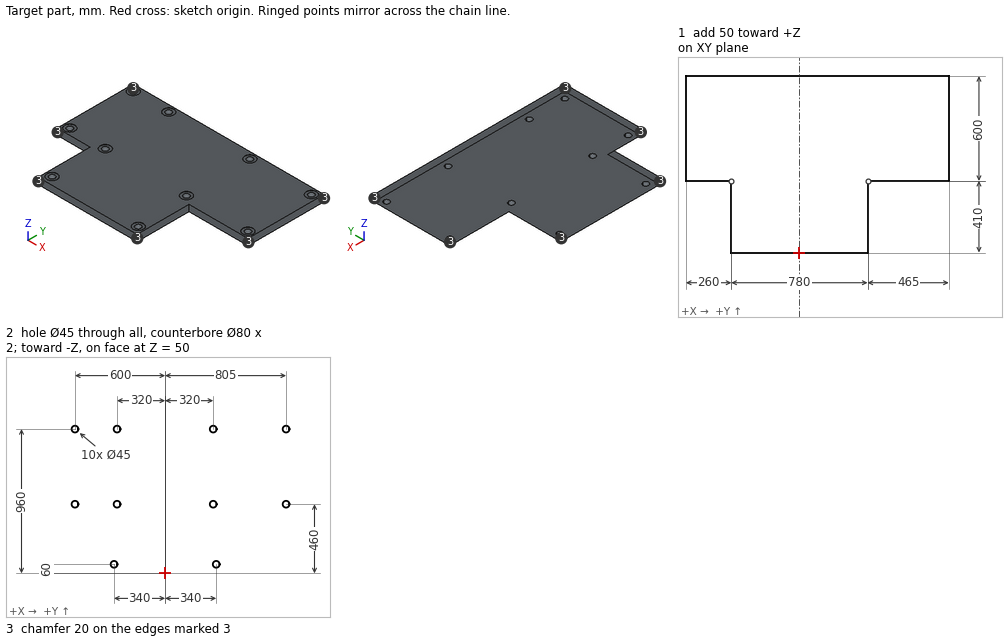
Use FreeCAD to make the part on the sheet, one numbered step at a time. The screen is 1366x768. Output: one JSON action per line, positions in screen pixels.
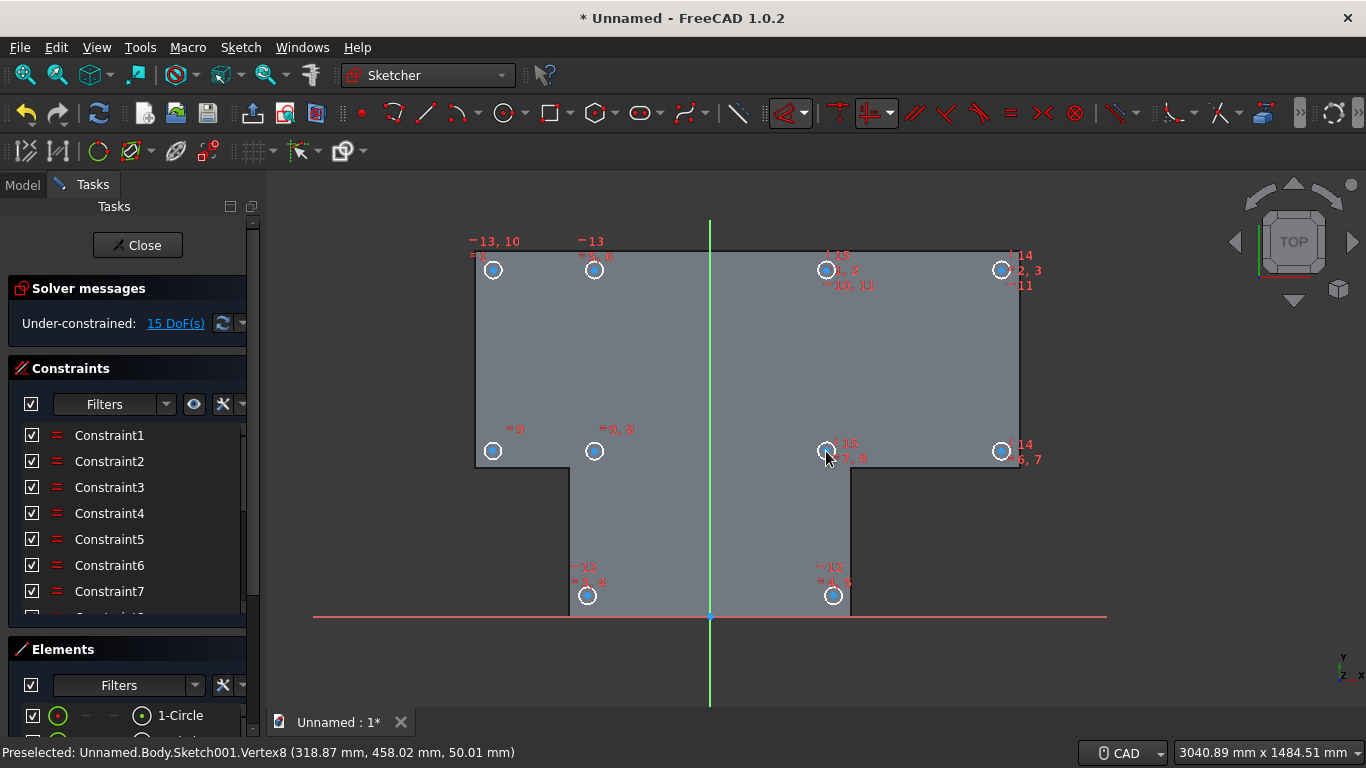
{"action": "left_click", "coordinate": [1002, 451]}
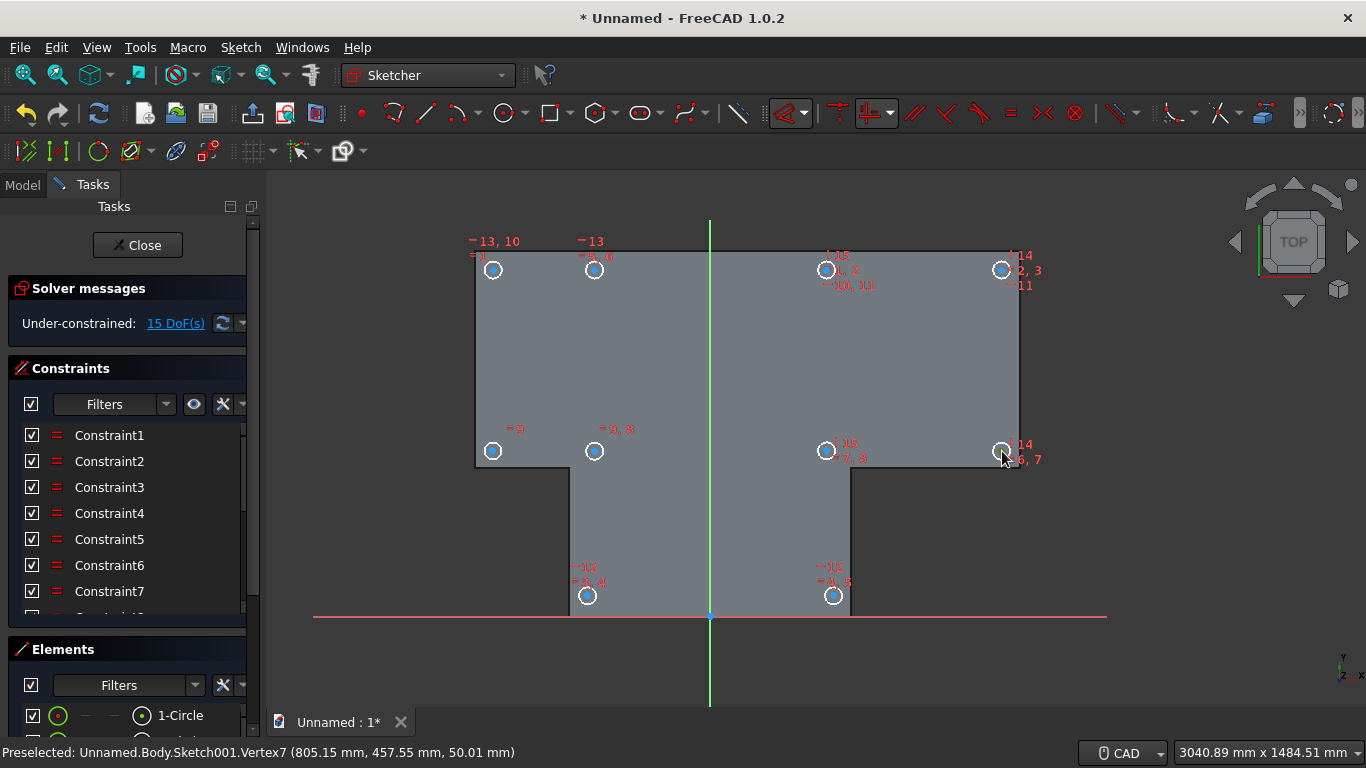
{"action": "left_click", "coordinate": [827, 451]}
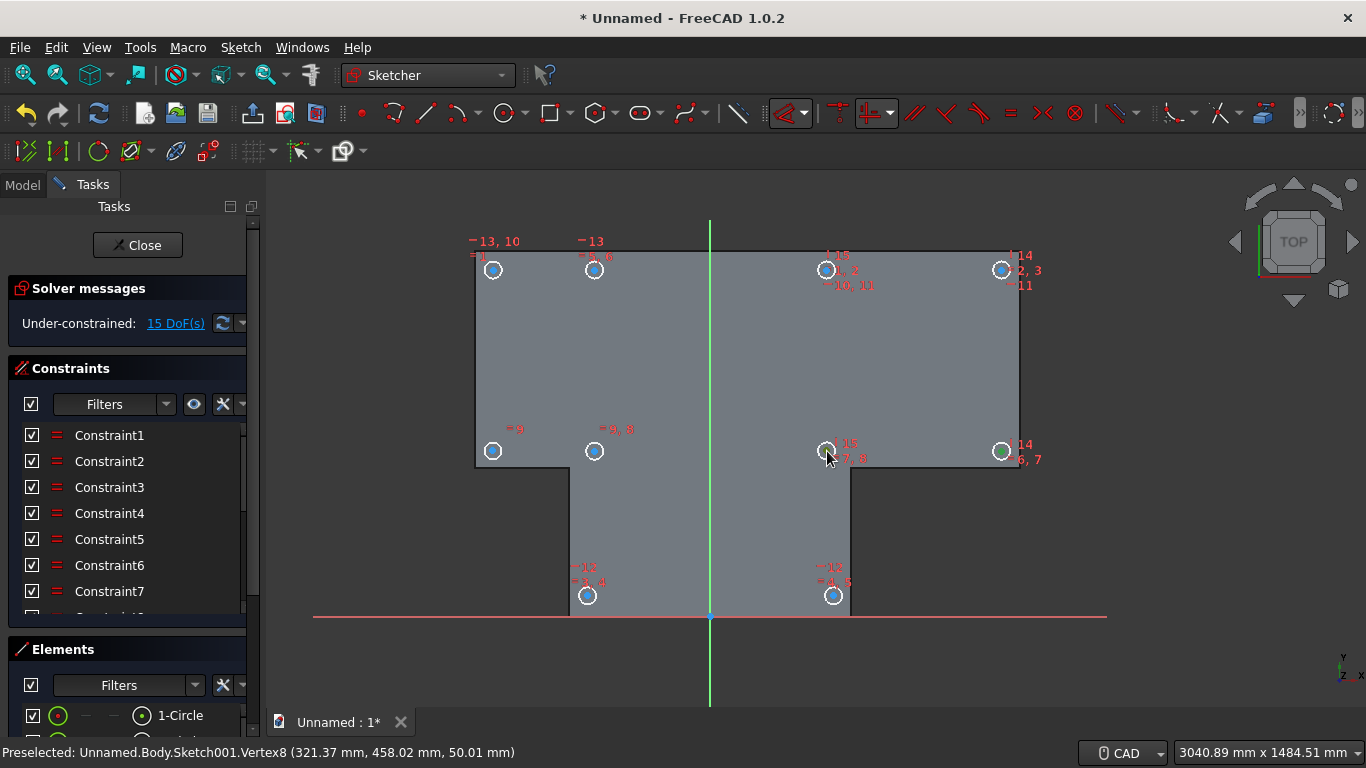
{"action": "left_click", "coordinate": [892, 114]}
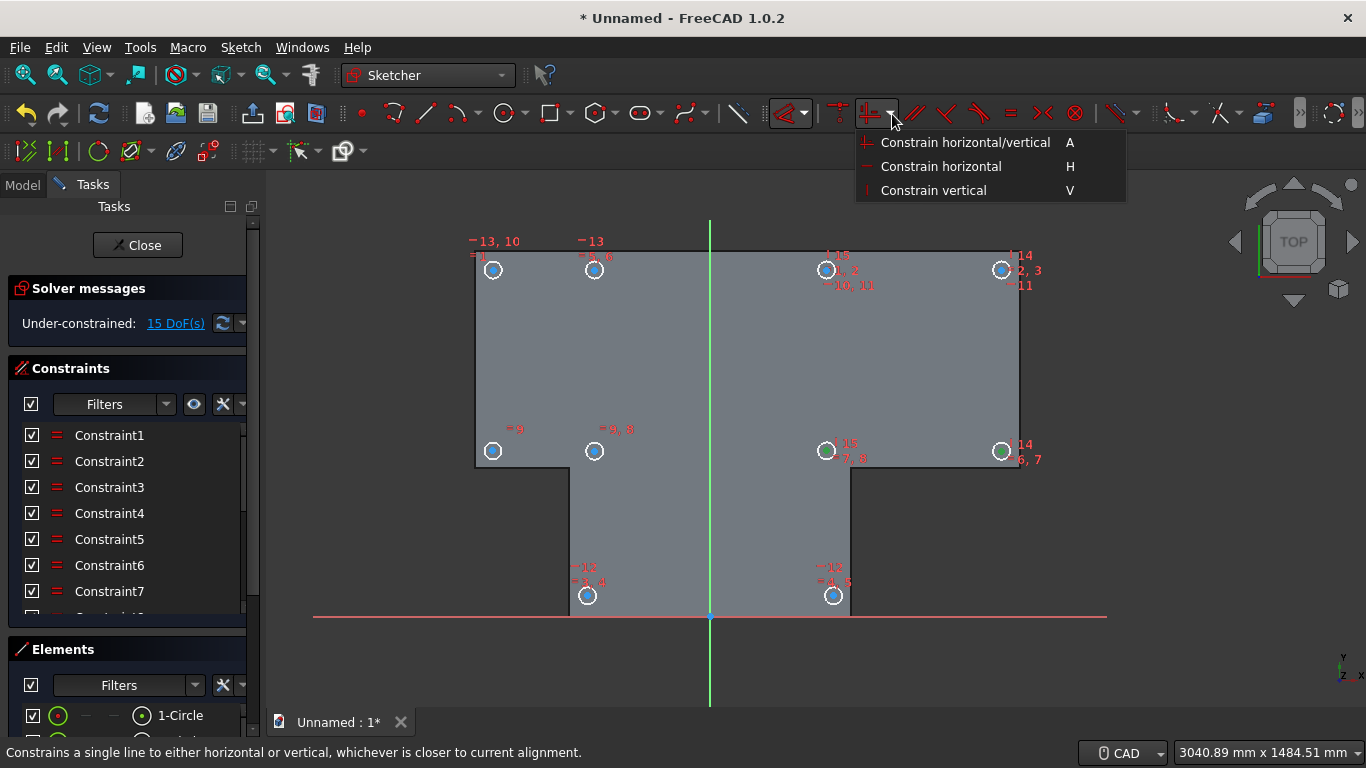
{"action": "left_click", "coordinate": [991, 166]}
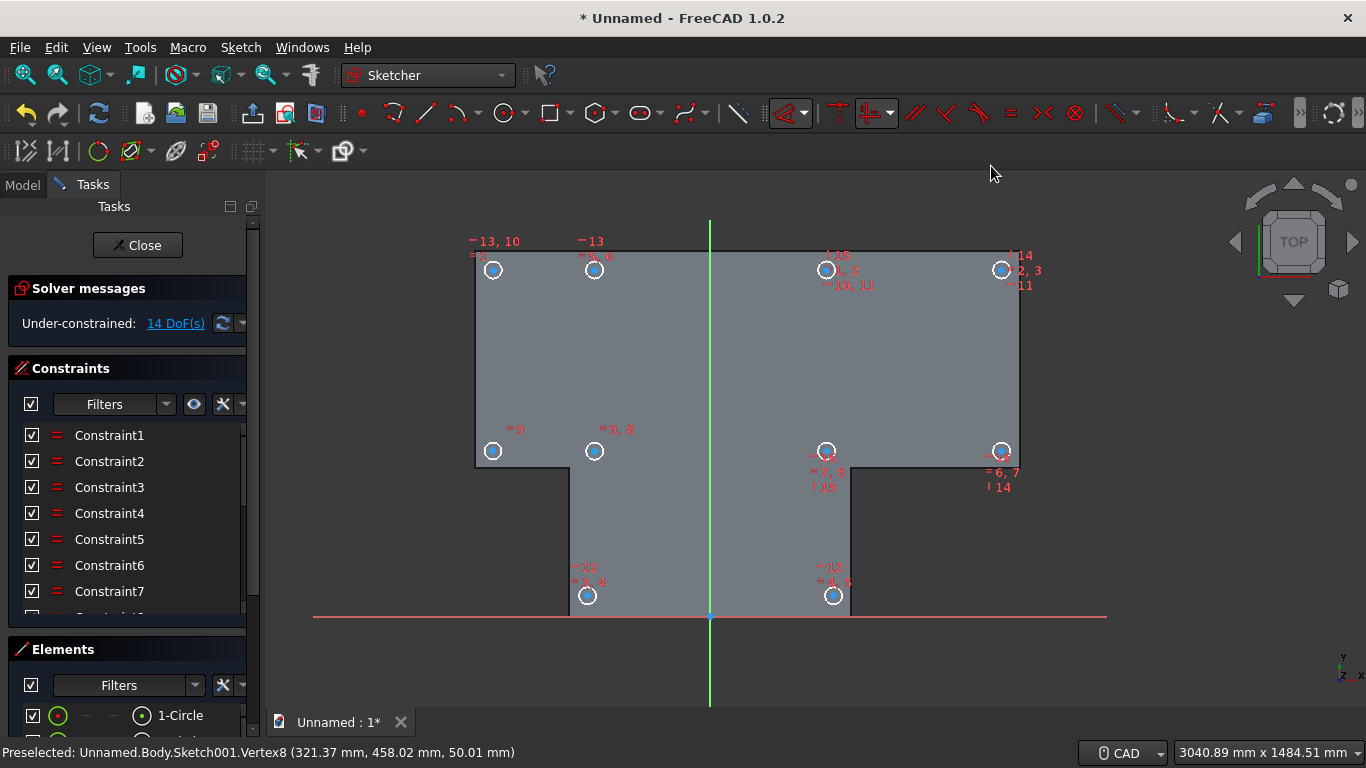
{"action": "left_click", "coordinate": [595, 270]}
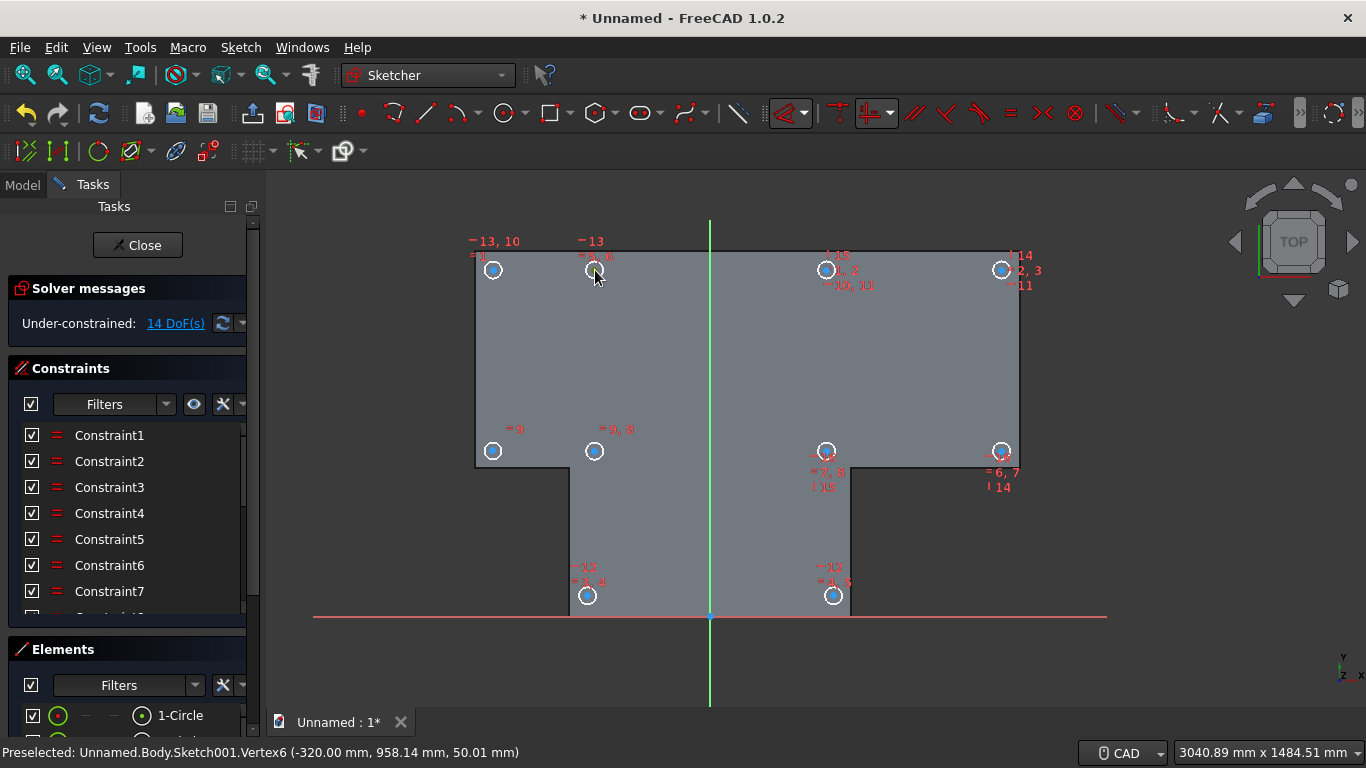
{"action": "left_click", "coordinate": [595, 451]}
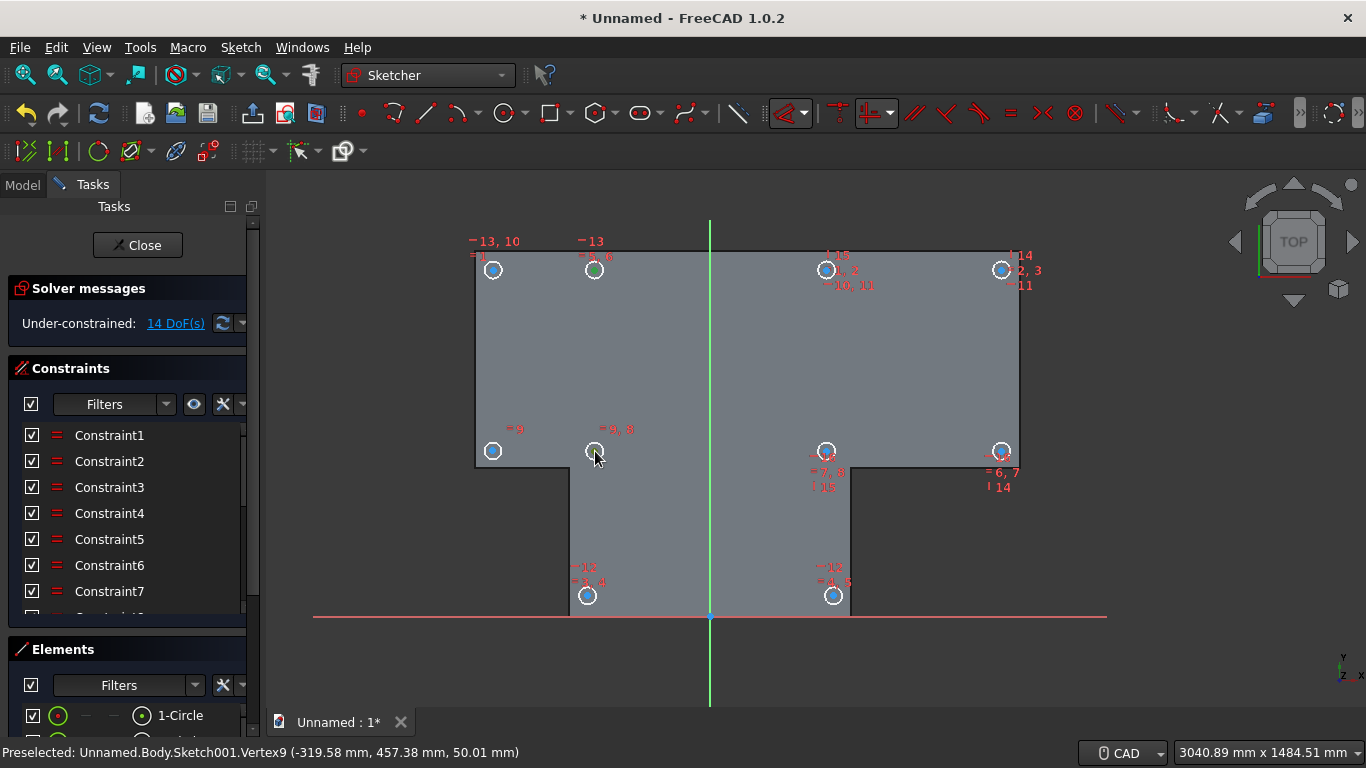
{"action": "key", "text": "v"}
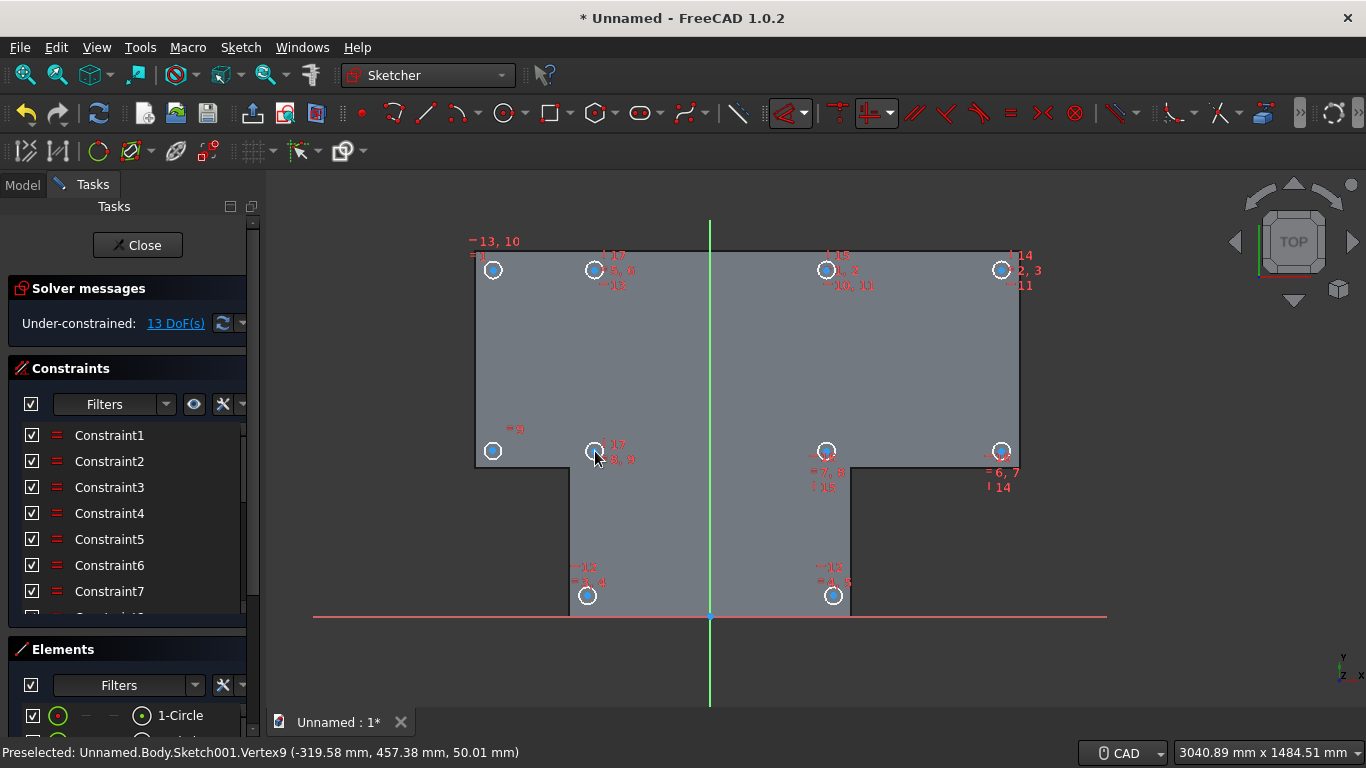
{"action": "left_click", "coordinate": [825, 449]}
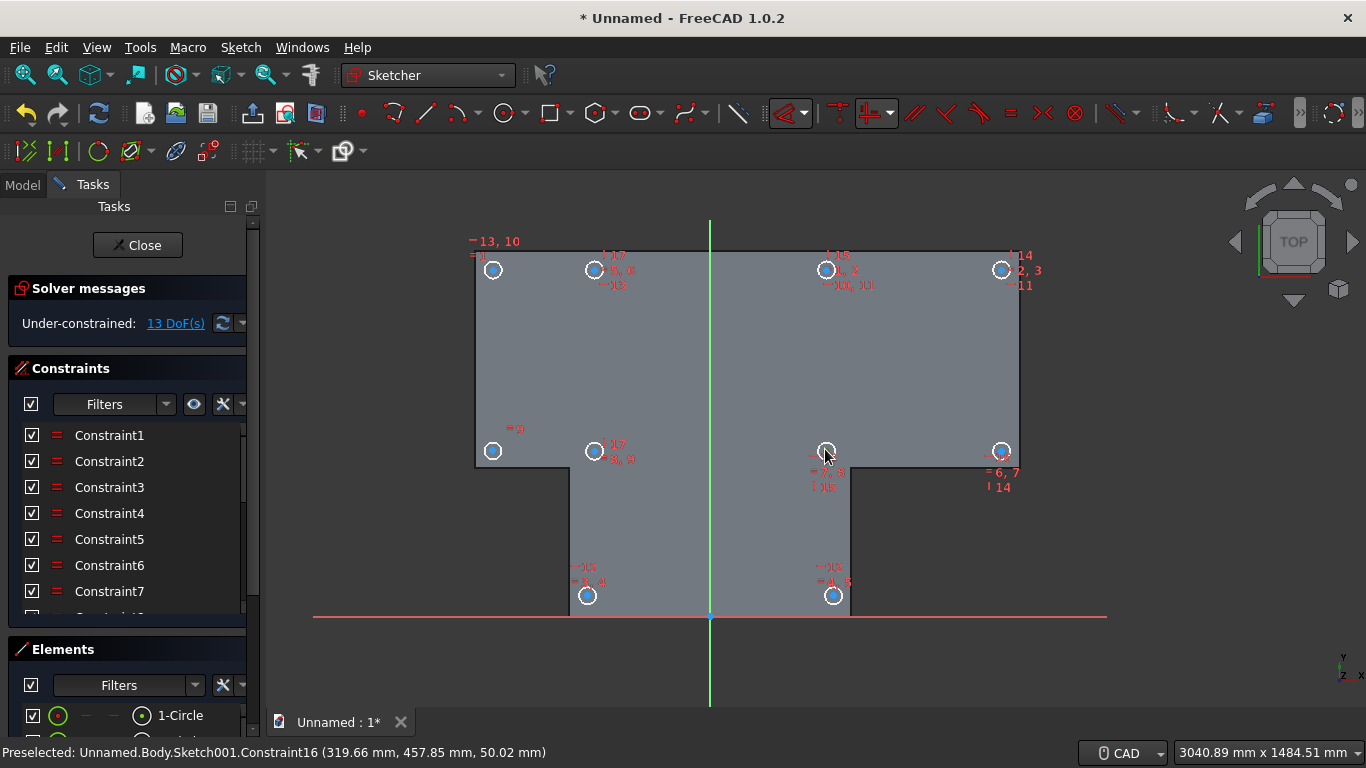
{"action": "left_click", "coordinate": [595, 451]}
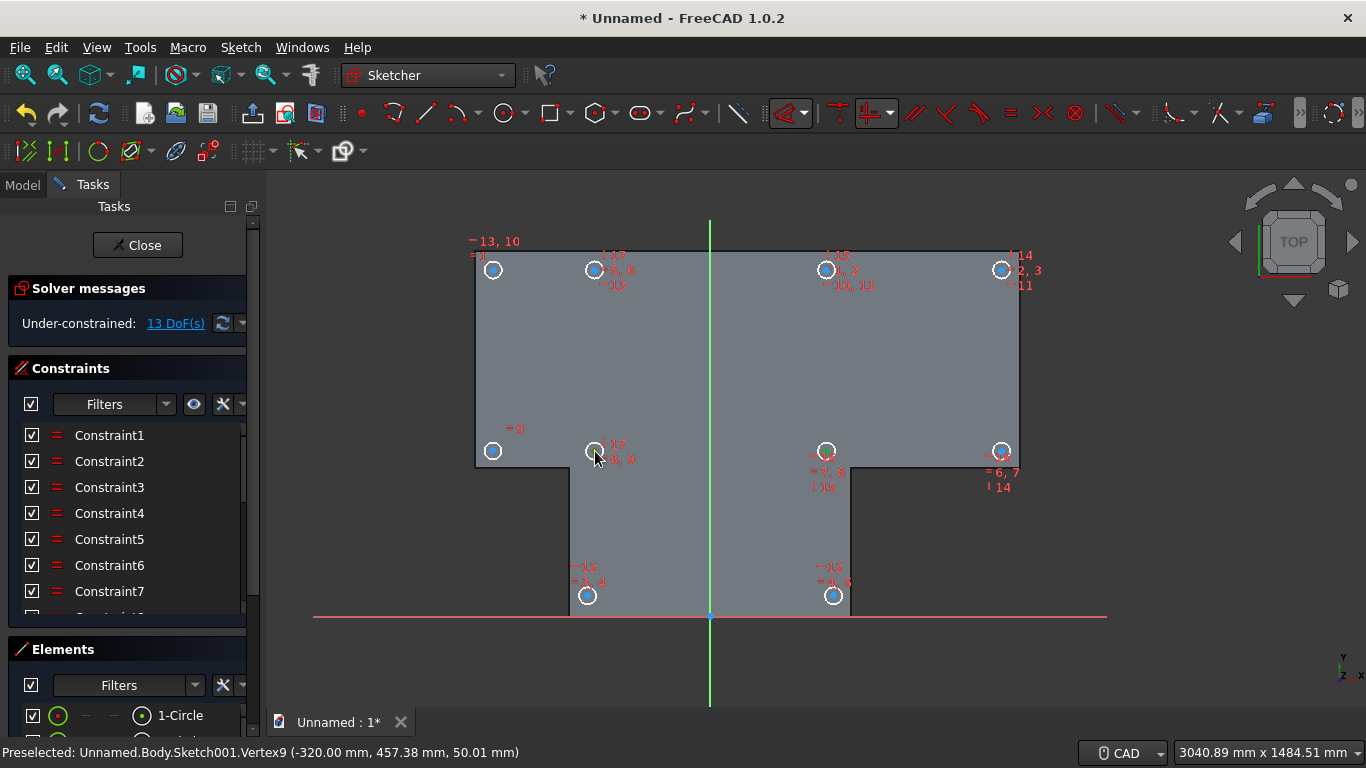
{"action": "left_click", "coordinate": [892, 114]}